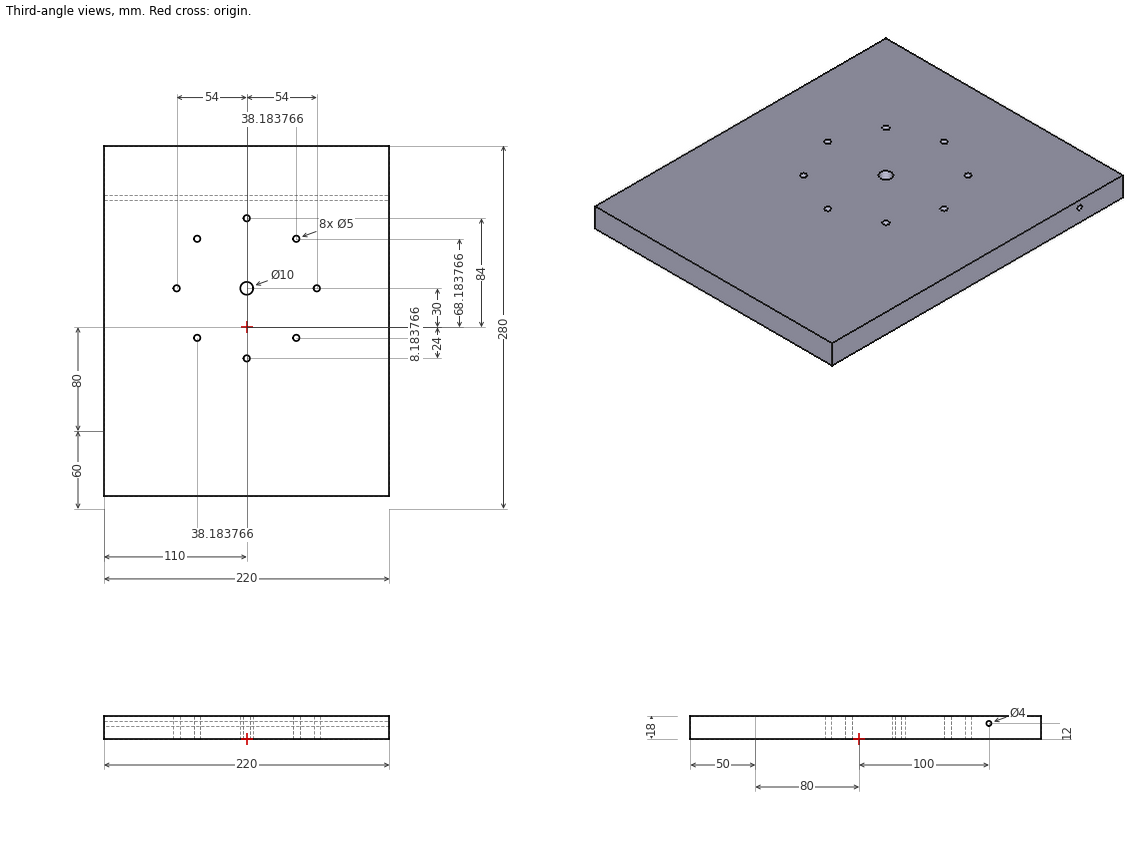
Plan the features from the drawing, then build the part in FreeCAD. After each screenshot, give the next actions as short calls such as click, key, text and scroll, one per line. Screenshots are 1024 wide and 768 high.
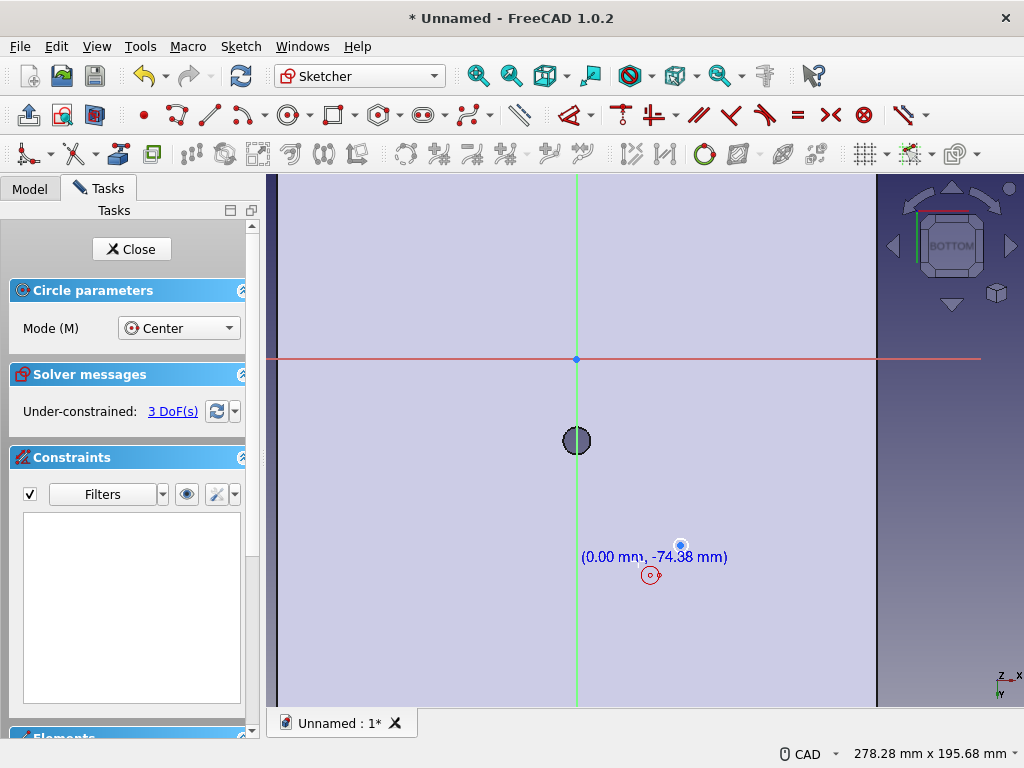
click(577, 588)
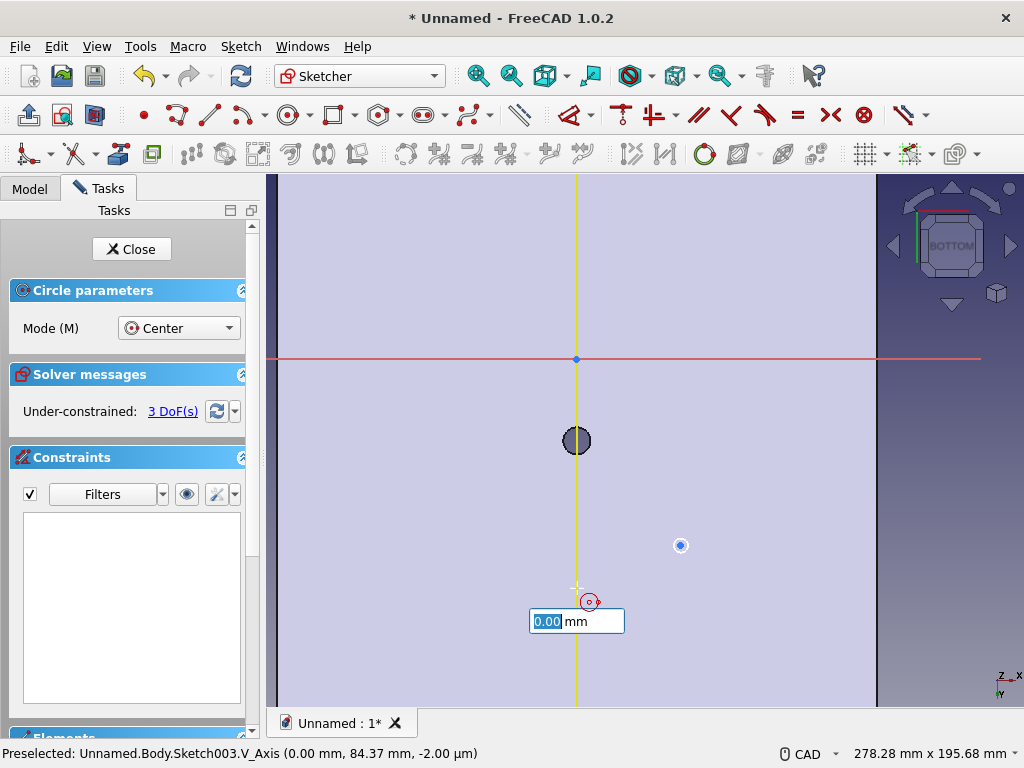
scroll(583, 586, up, 5)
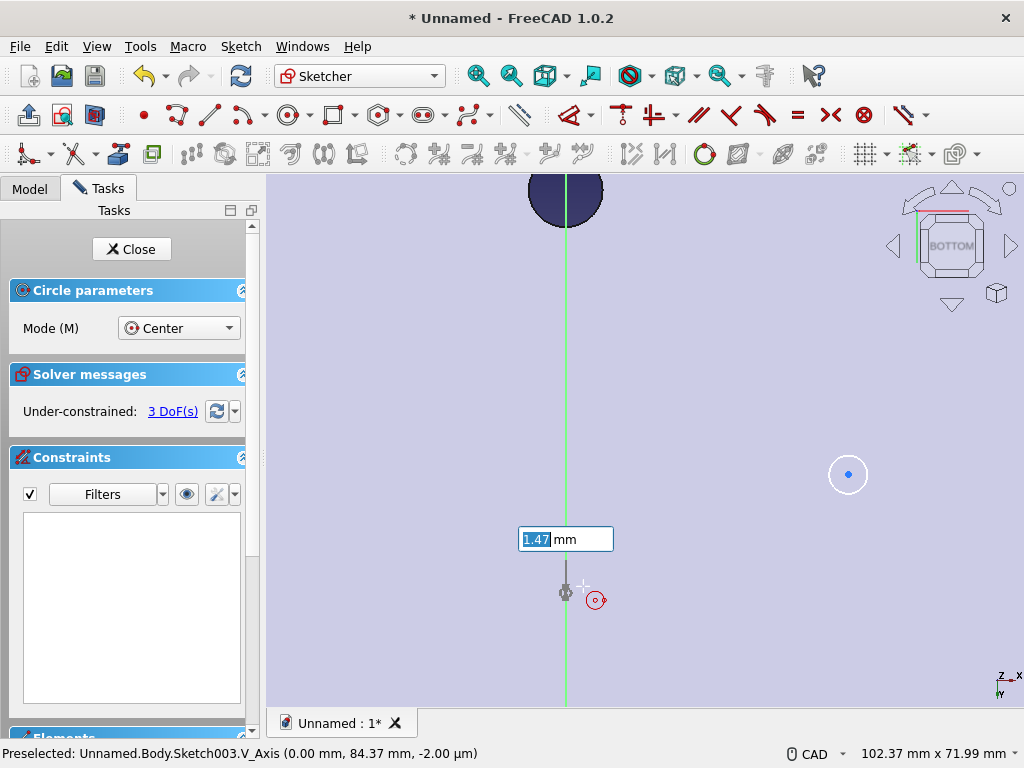
click(583, 584)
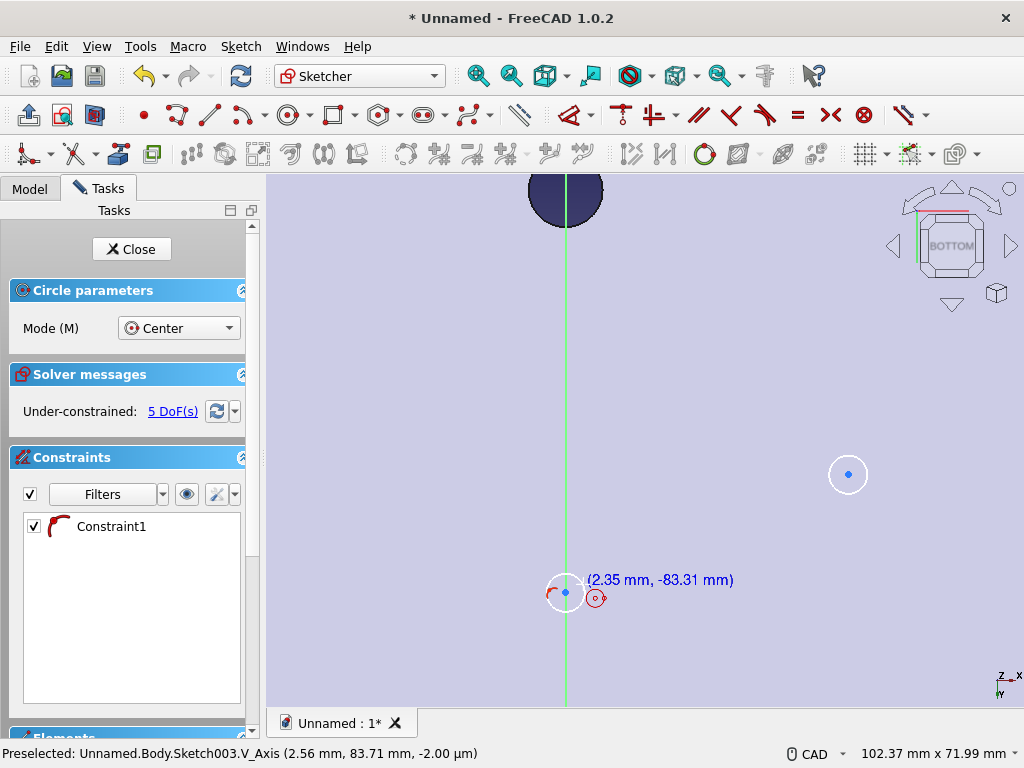
scroll(583, 586, down, 5)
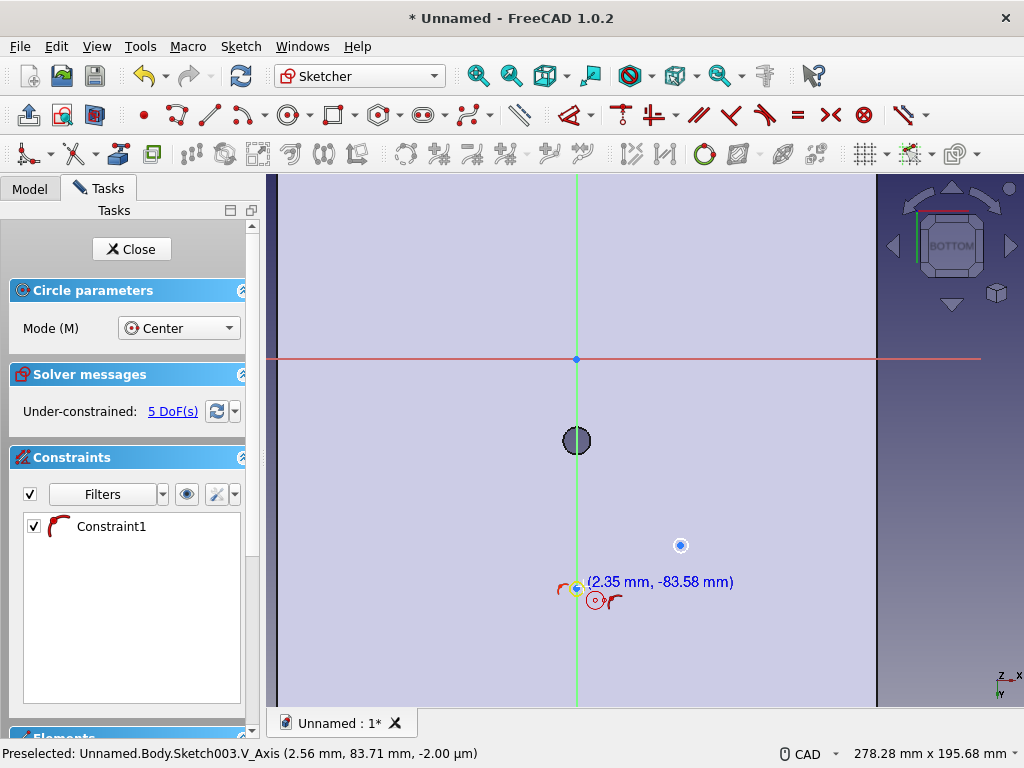
scroll(724, 441, up, 7)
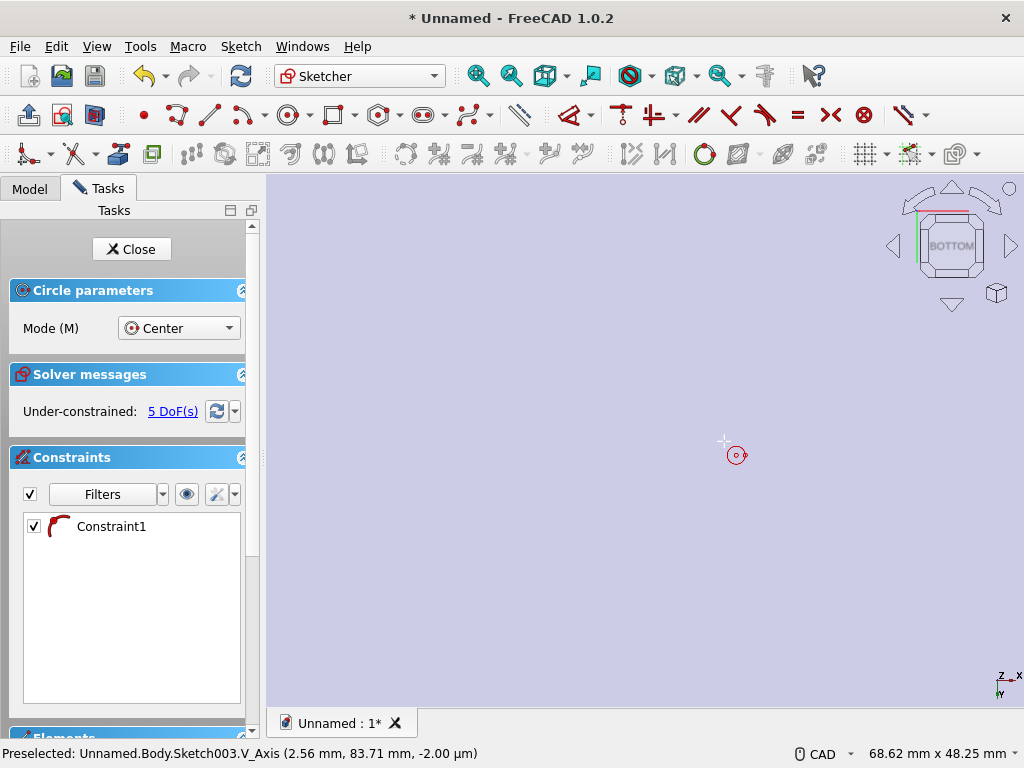
scroll(724, 441, down, 7)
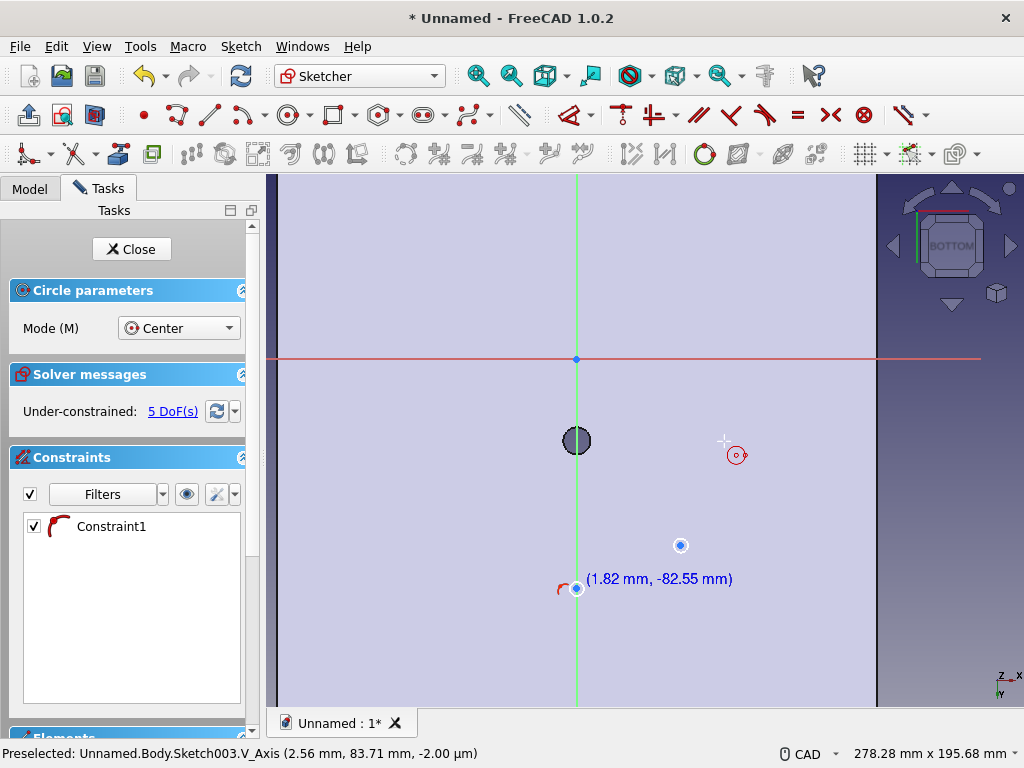
click(724, 441)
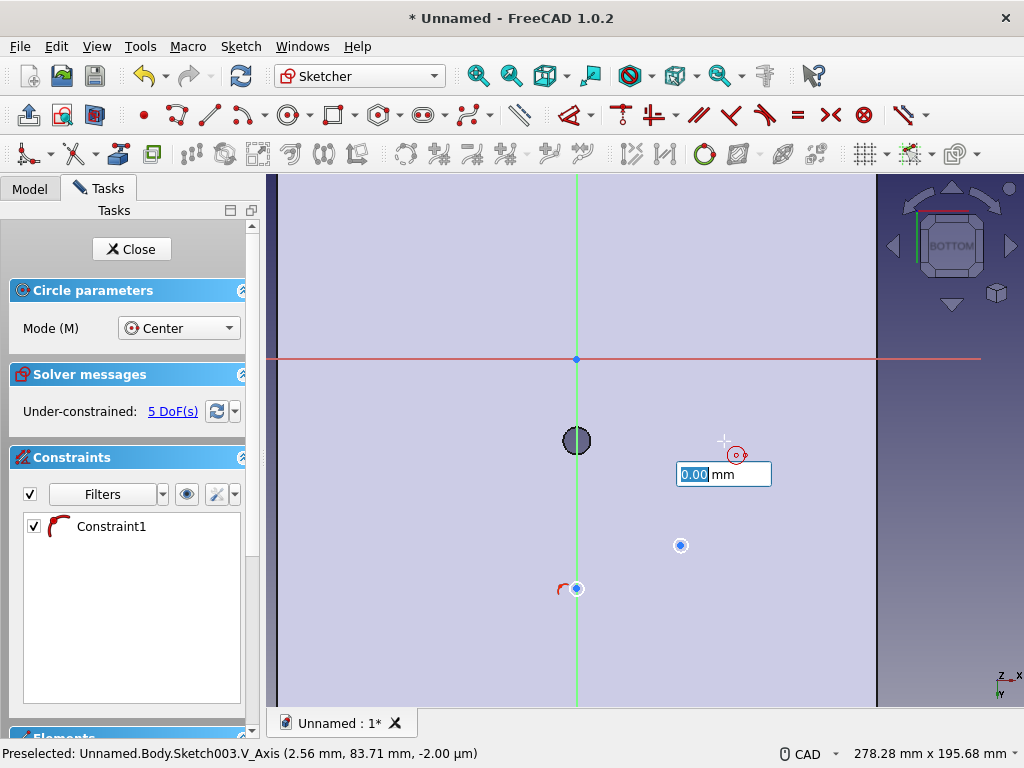
scroll(729, 436, up, 5)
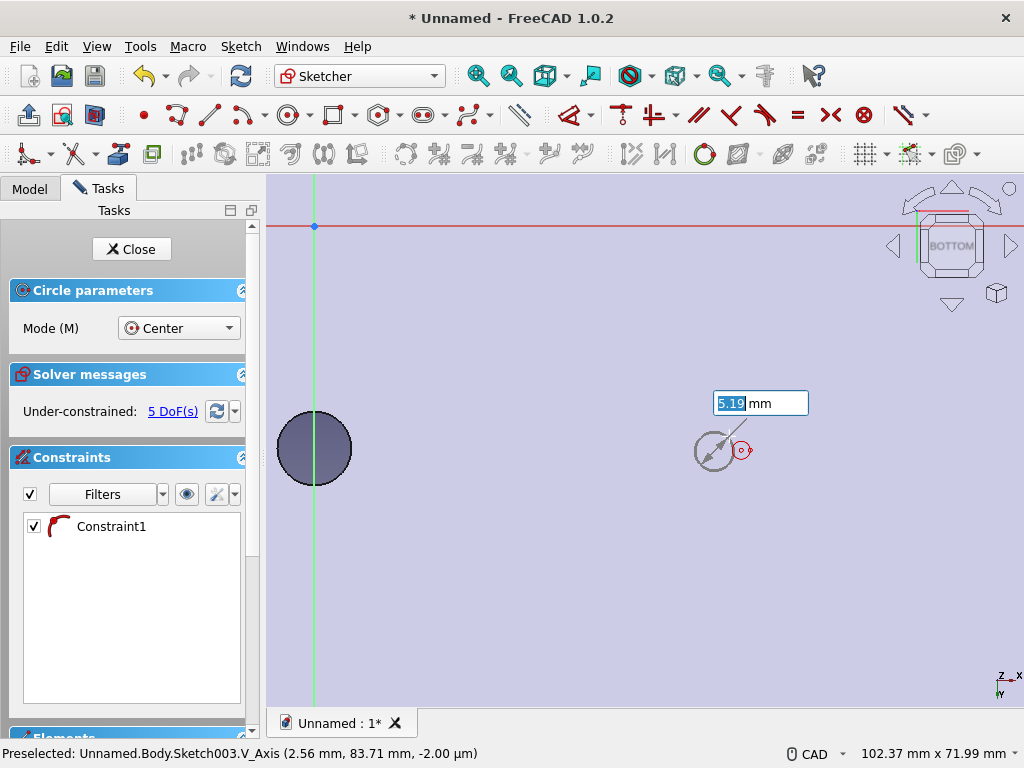
click(727, 435)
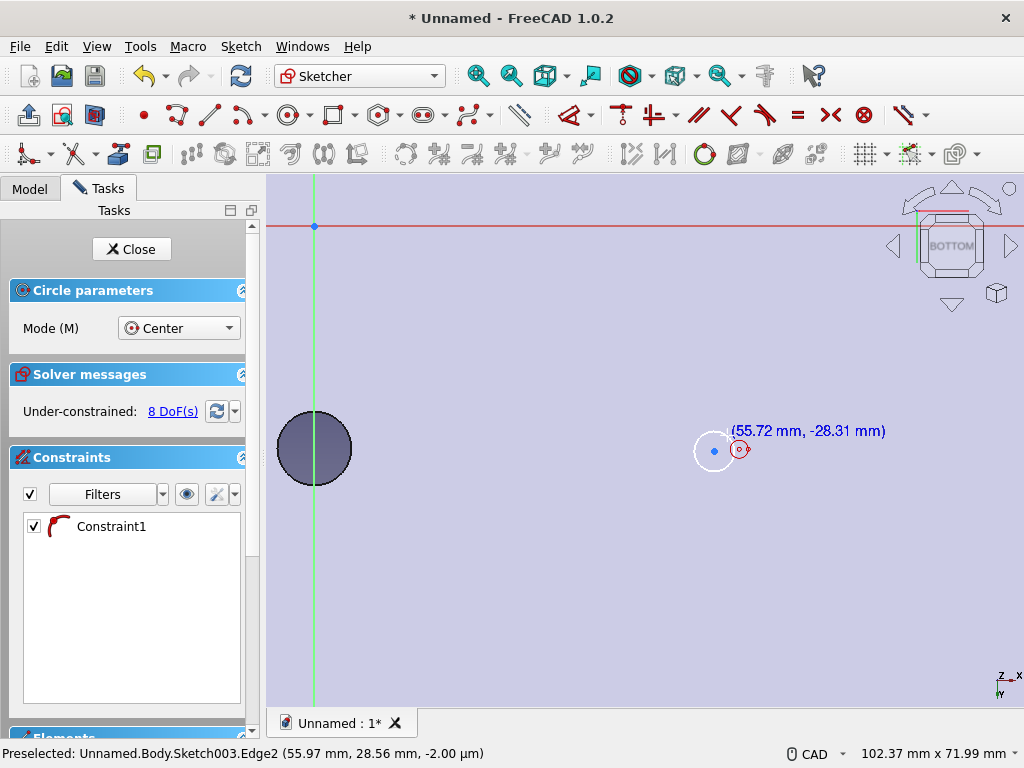
scroll(729, 436, down, 5)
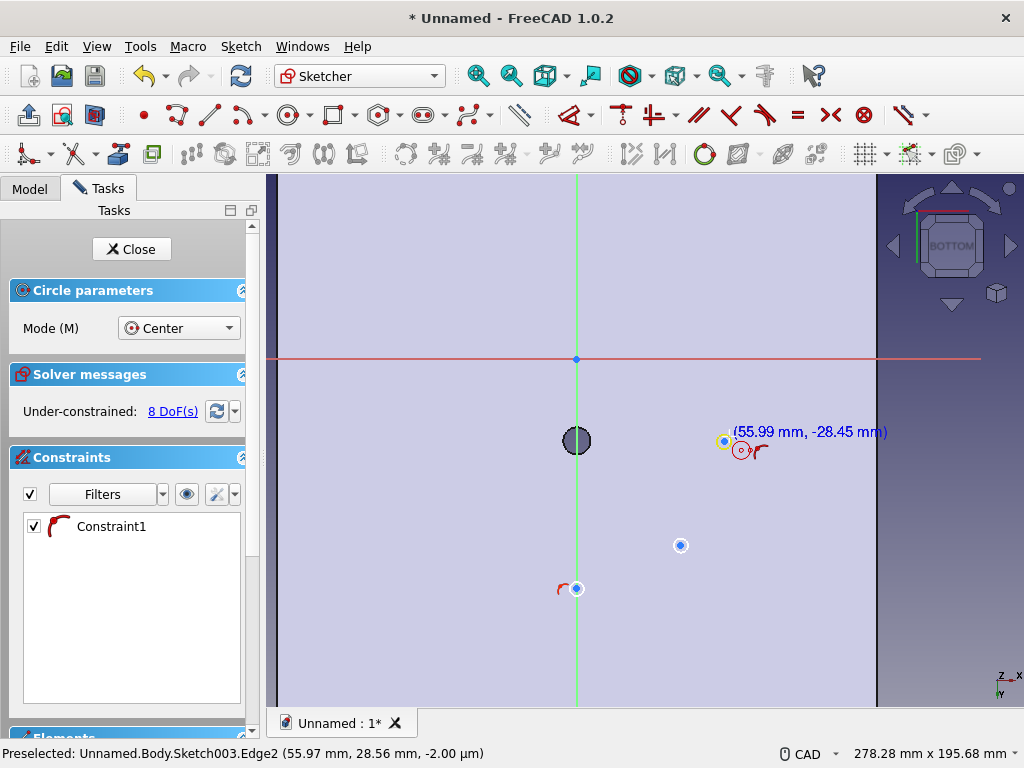
scroll(681, 337, up, 7)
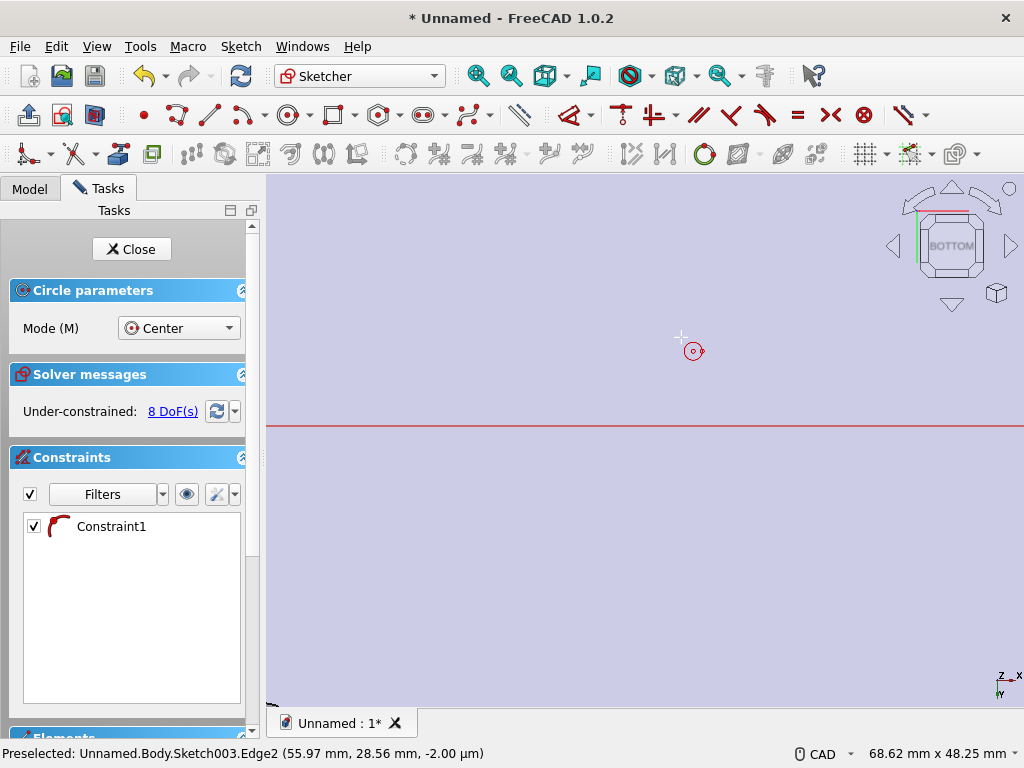
scroll(681, 337, down, 7)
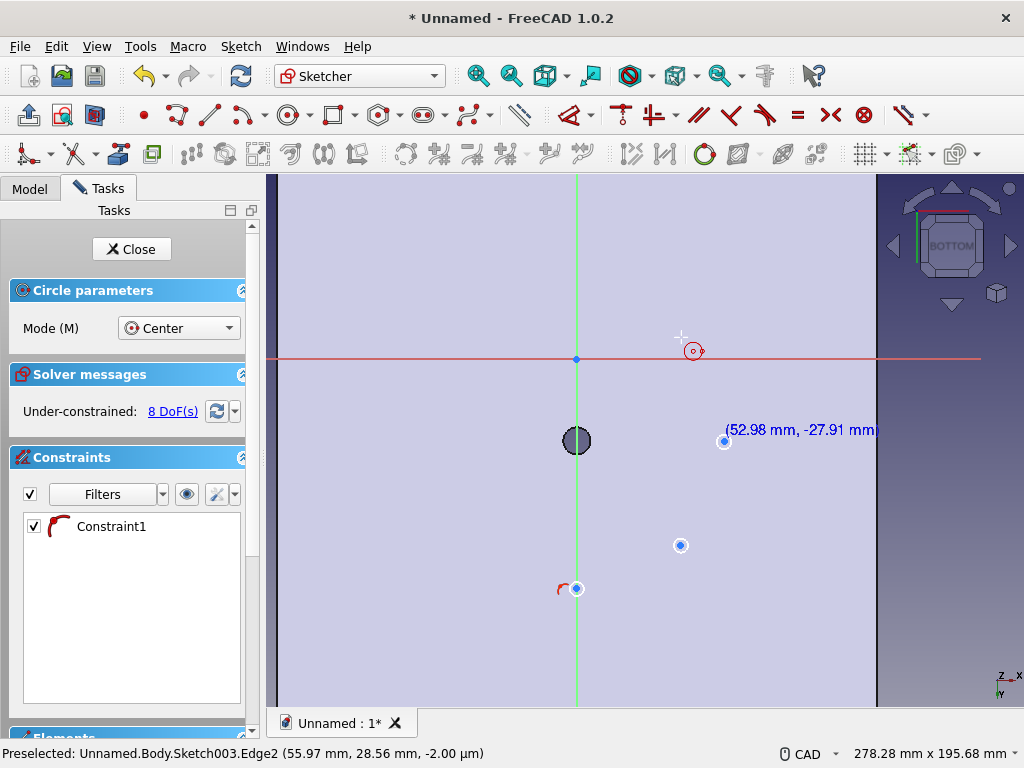
click(681, 337)